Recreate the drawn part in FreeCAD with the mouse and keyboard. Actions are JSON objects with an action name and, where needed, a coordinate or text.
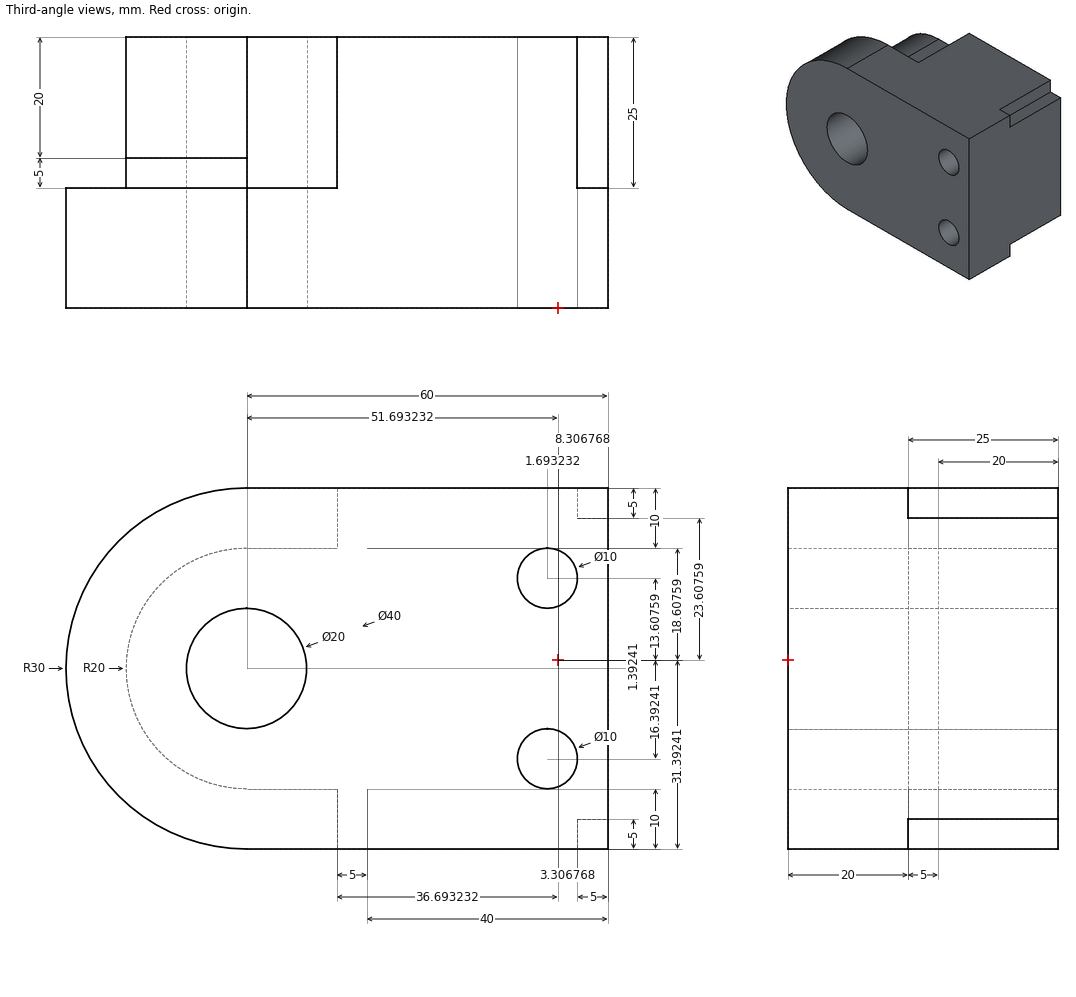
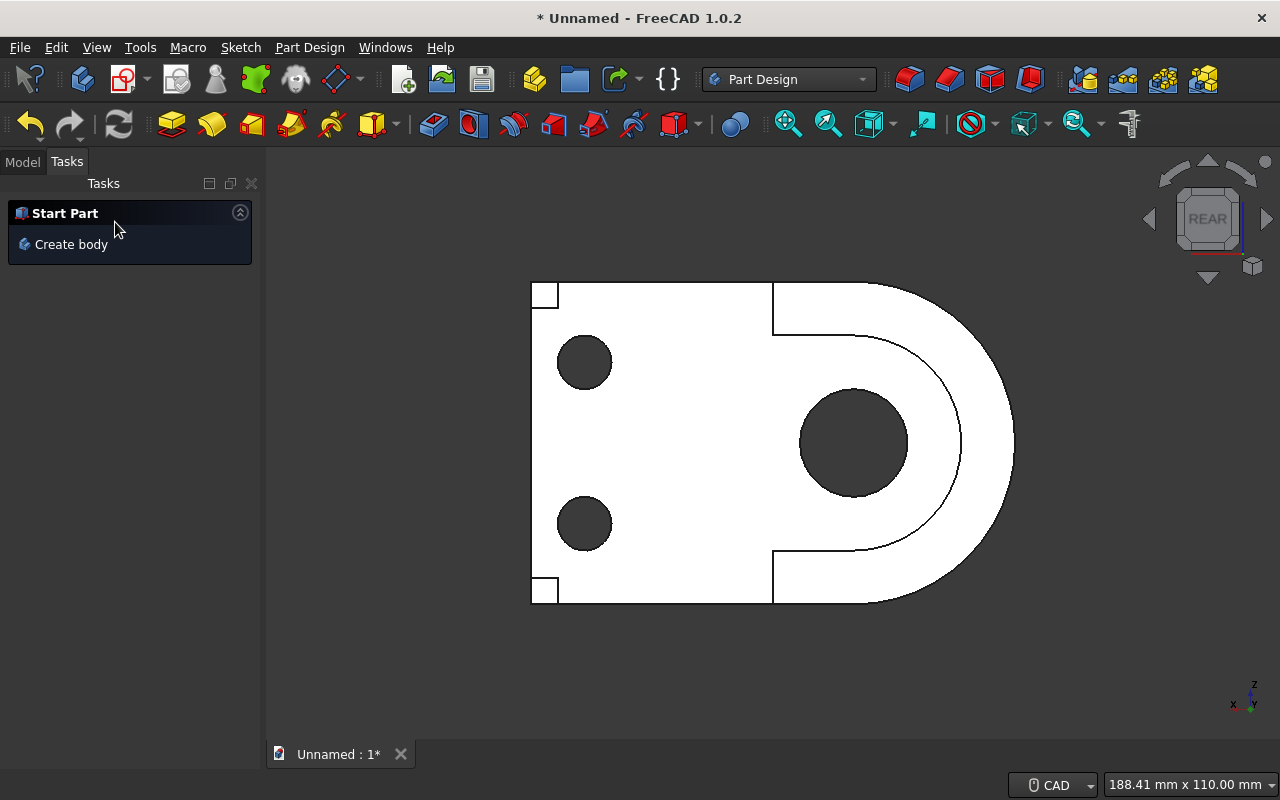
{"action": "key", "text": "0"}